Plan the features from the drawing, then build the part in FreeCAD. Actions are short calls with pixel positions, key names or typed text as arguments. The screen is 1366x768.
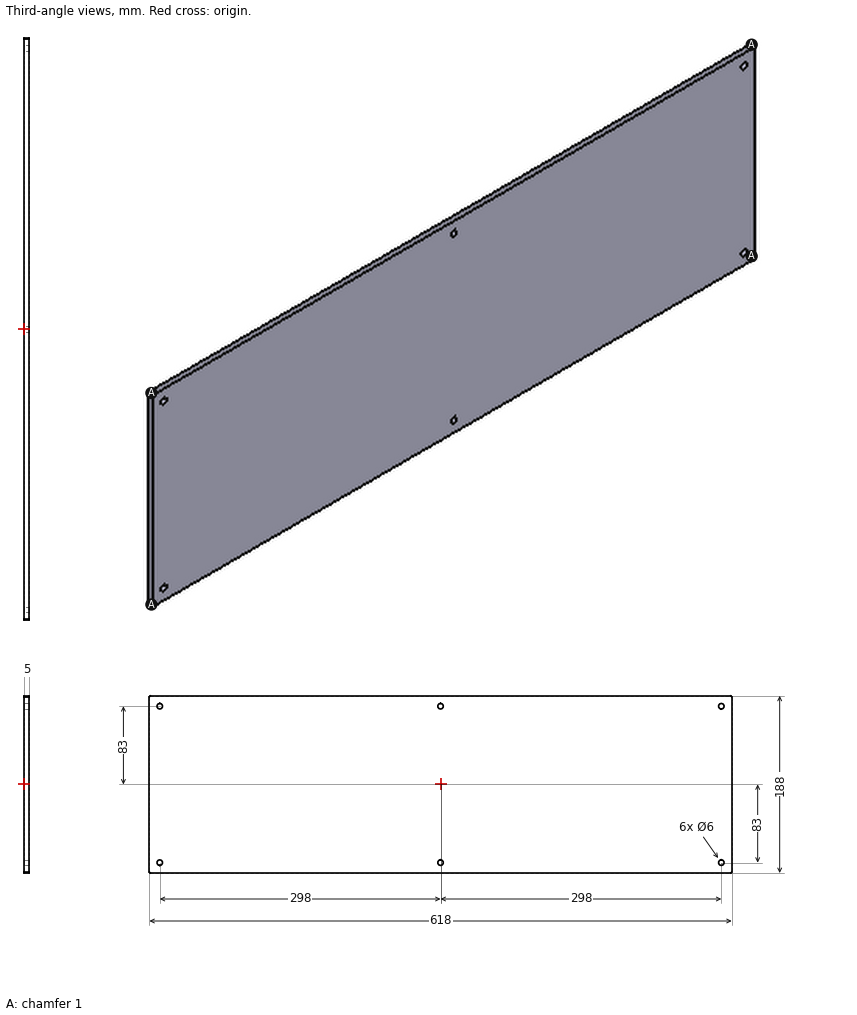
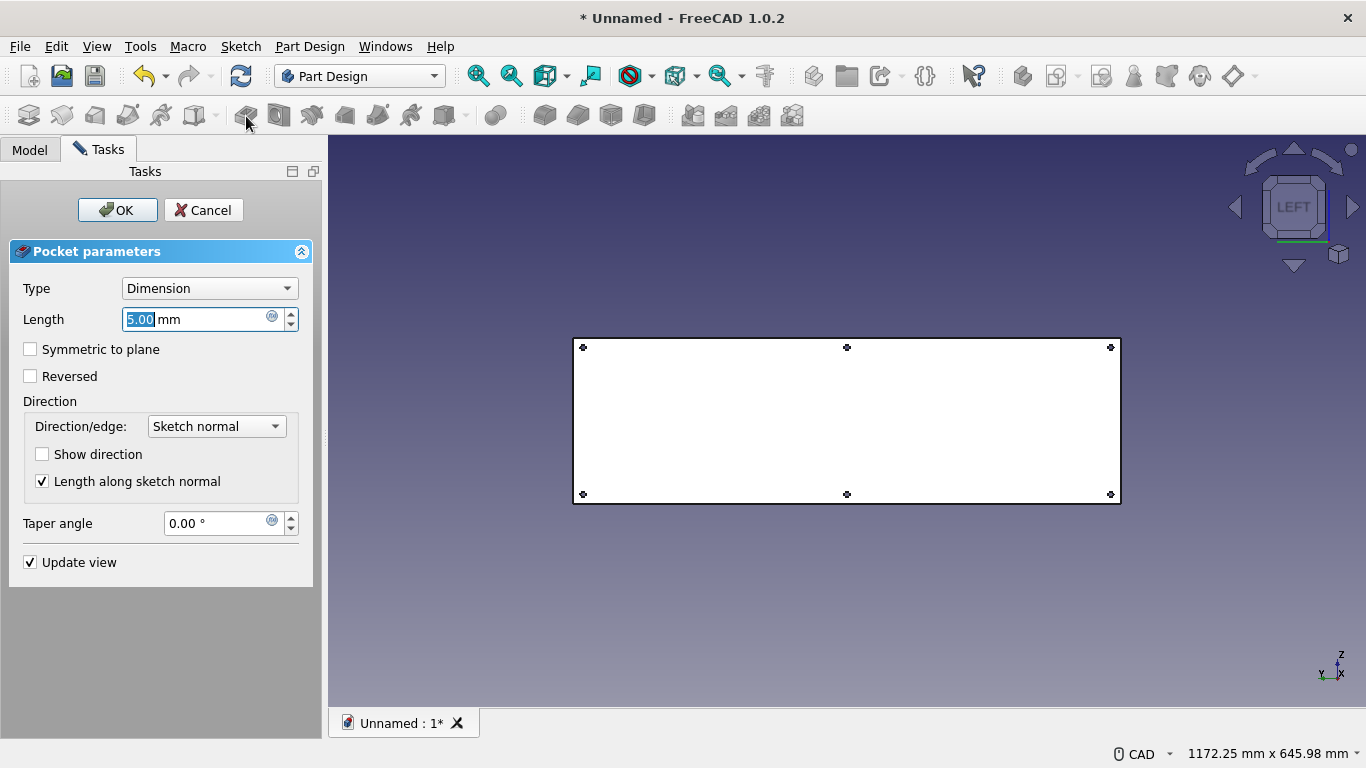
click(210, 288)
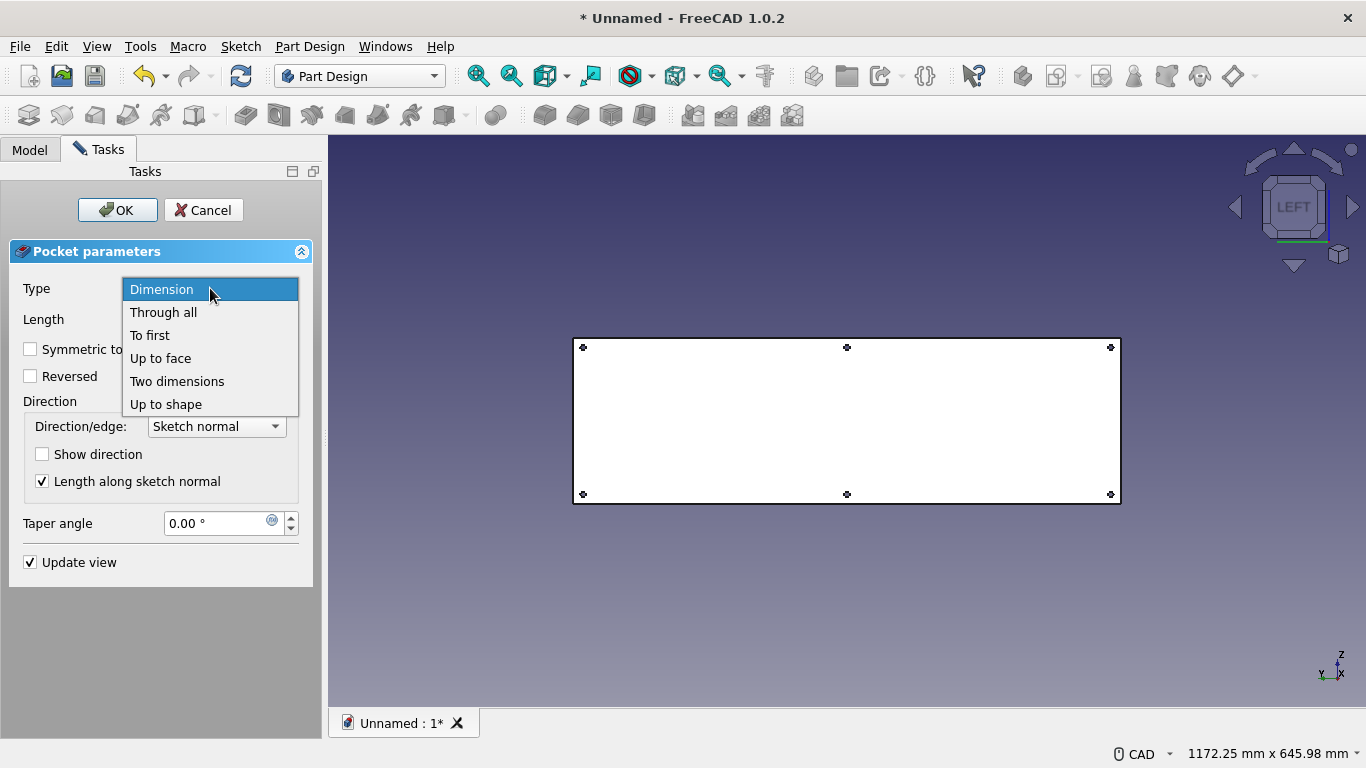
click(208, 312)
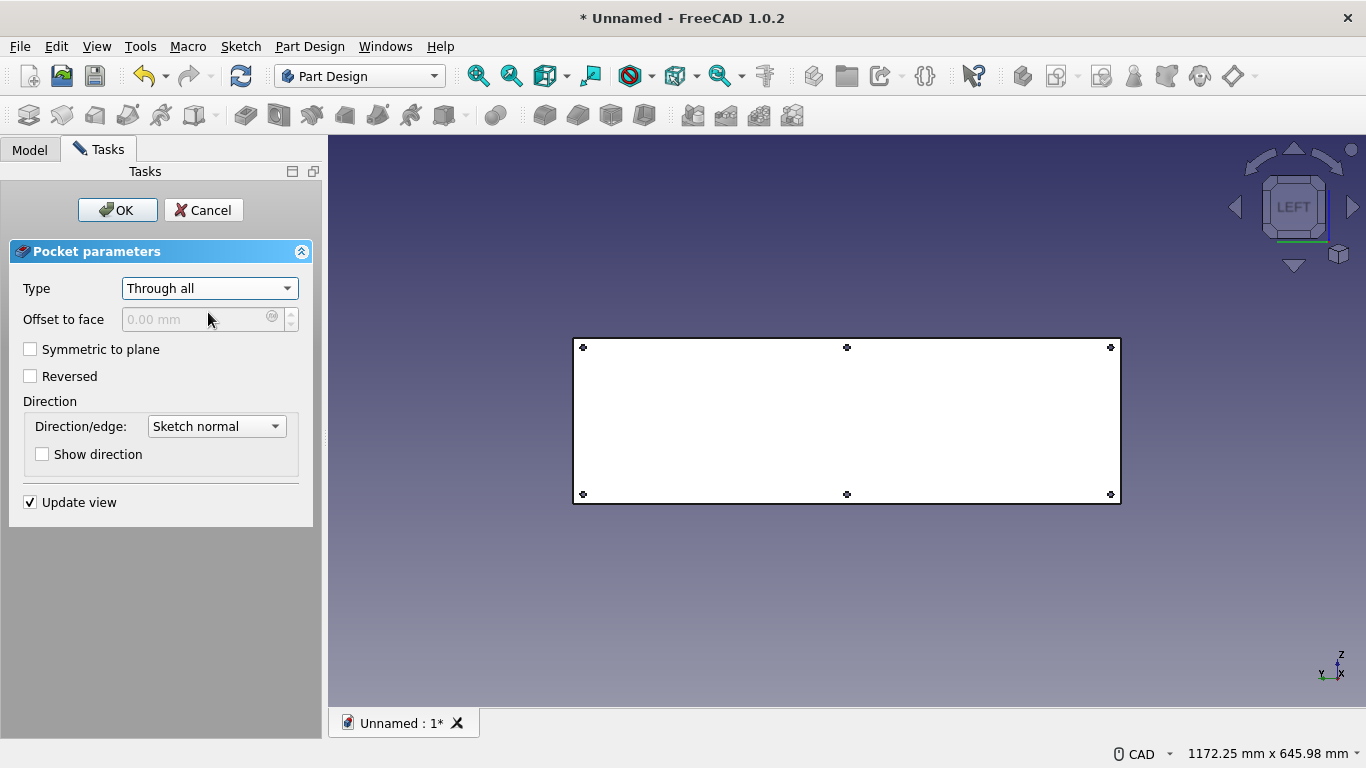
click(118, 210)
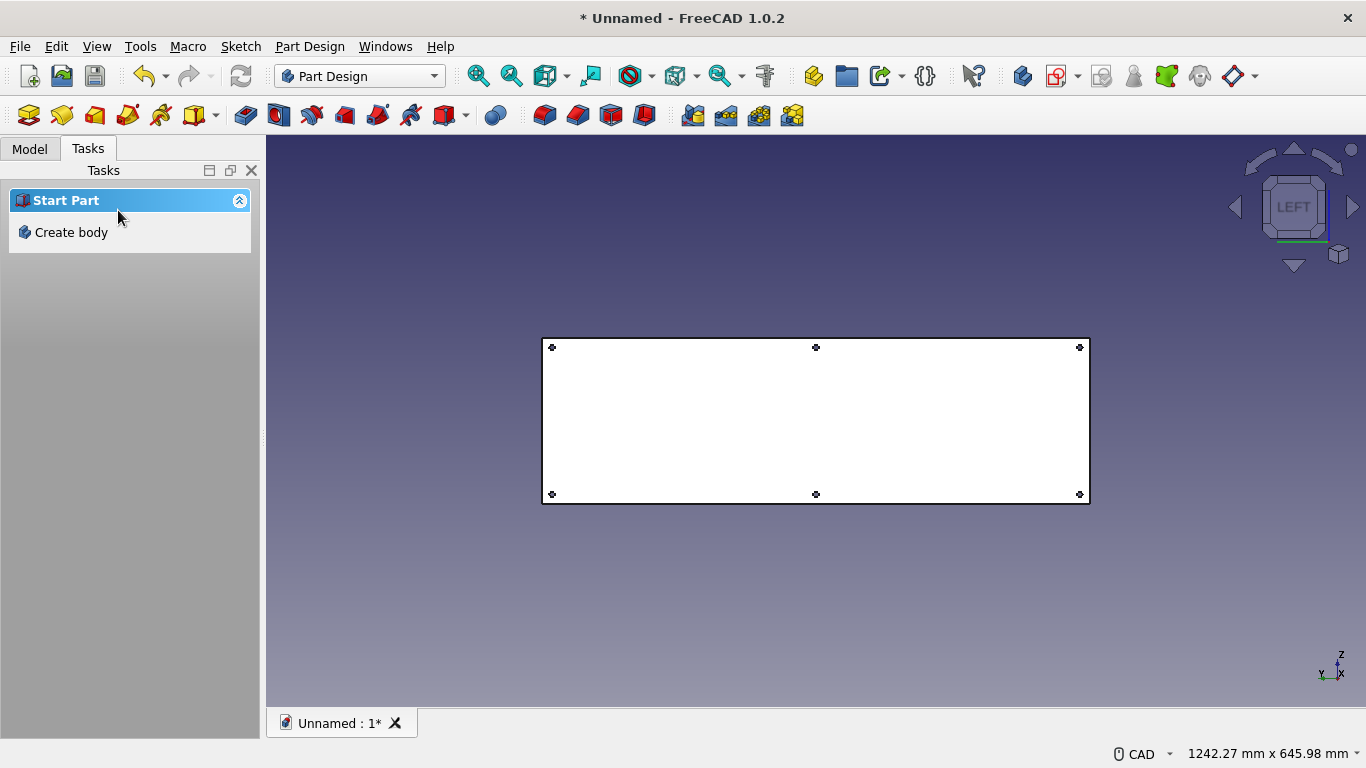
key(0)